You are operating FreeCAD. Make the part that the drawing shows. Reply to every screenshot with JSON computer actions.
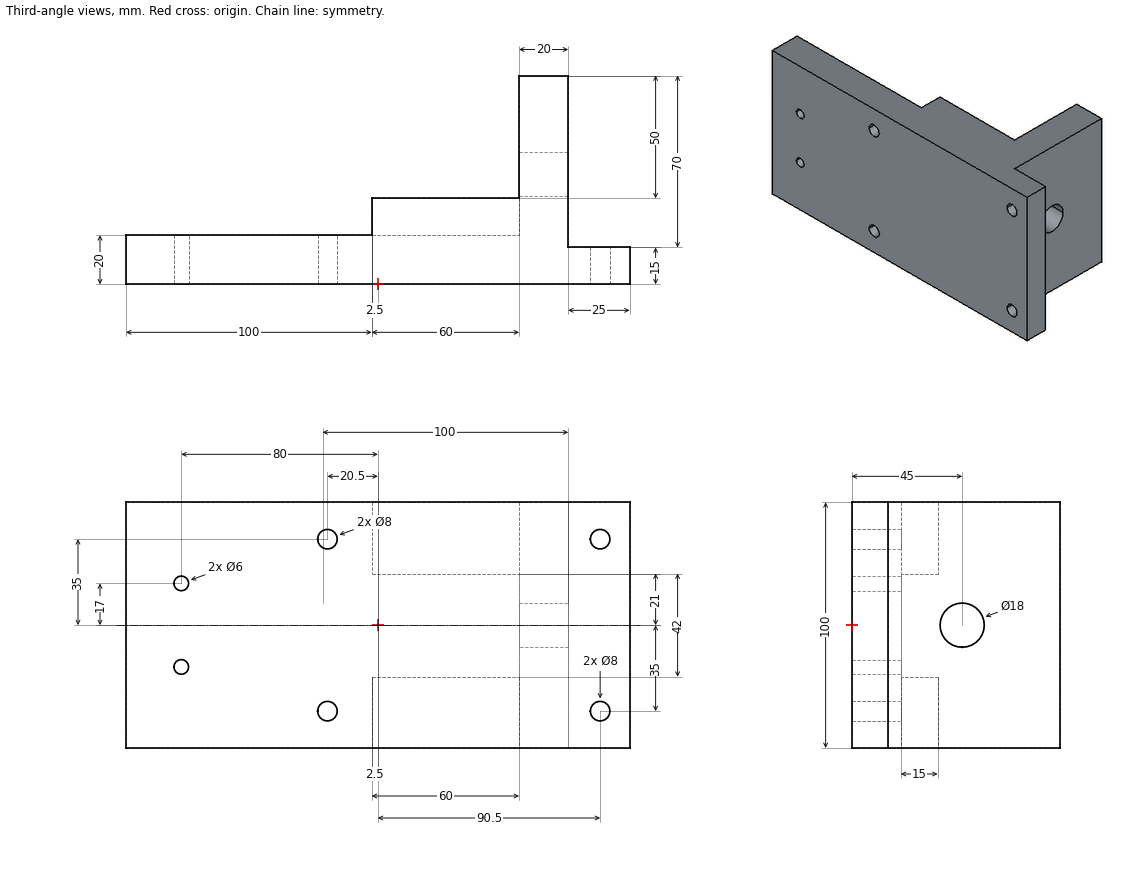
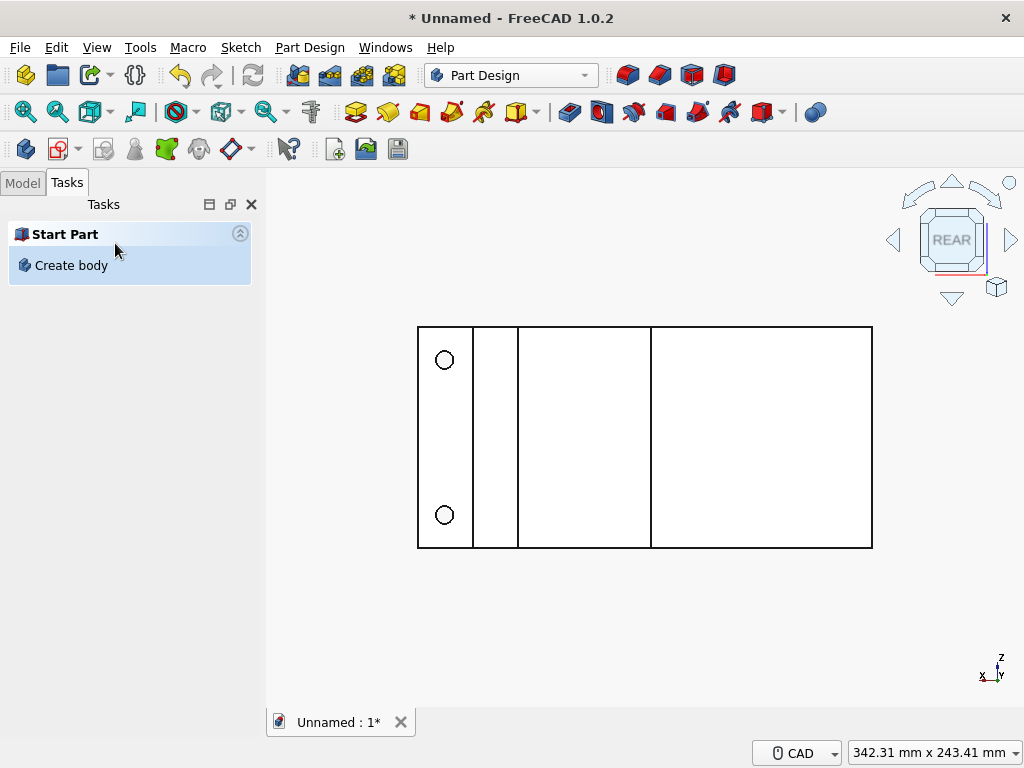
{"action": "left_click", "coordinate": [584, 405]}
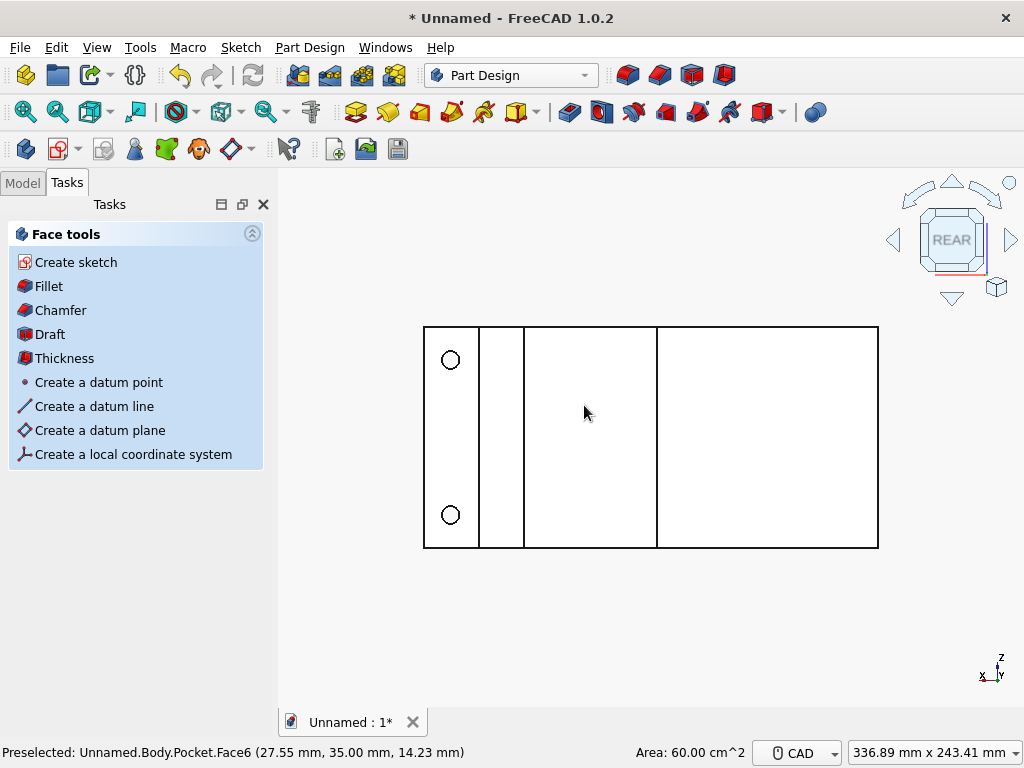
{"action": "left_click", "coordinate": [58, 150]}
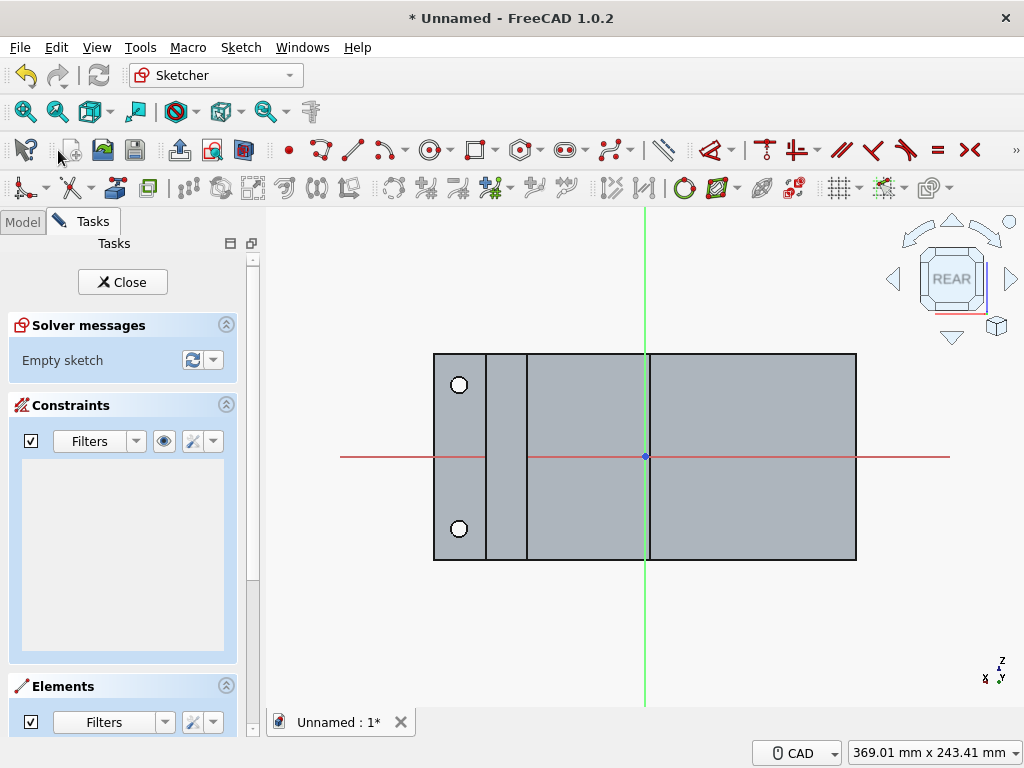
{"action": "left_click", "coordinate": [244, 150]}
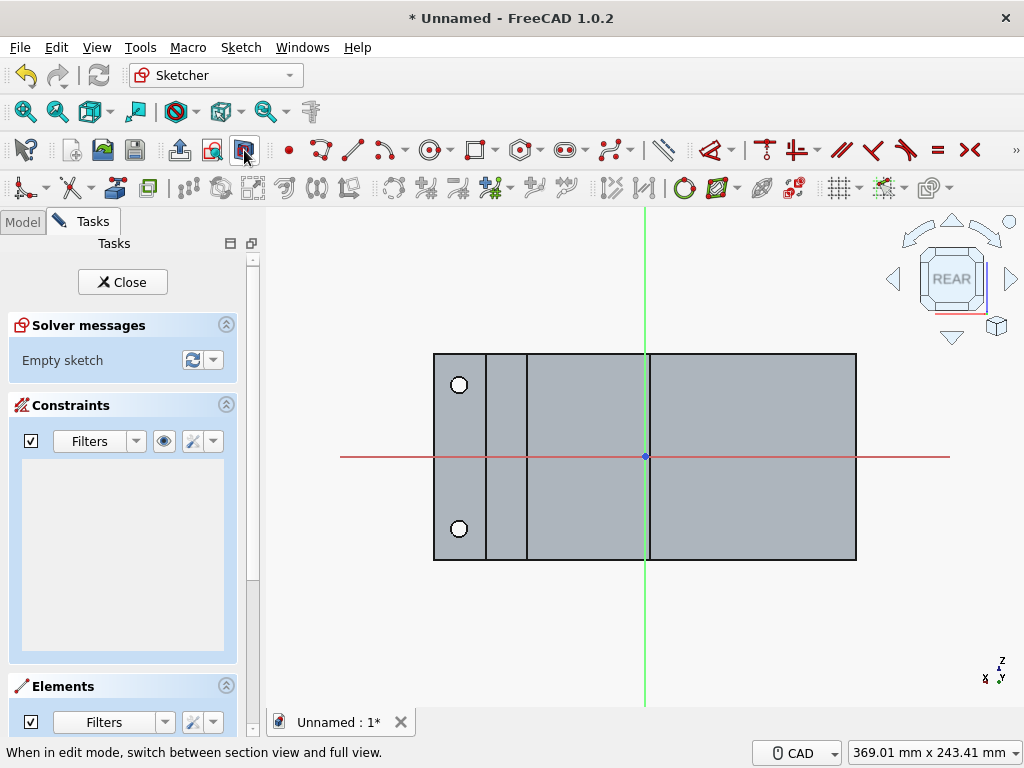
{"action": "scroll", "coordinate": [594, 457], "scroll_direction": "up", "scroll_amount": 6}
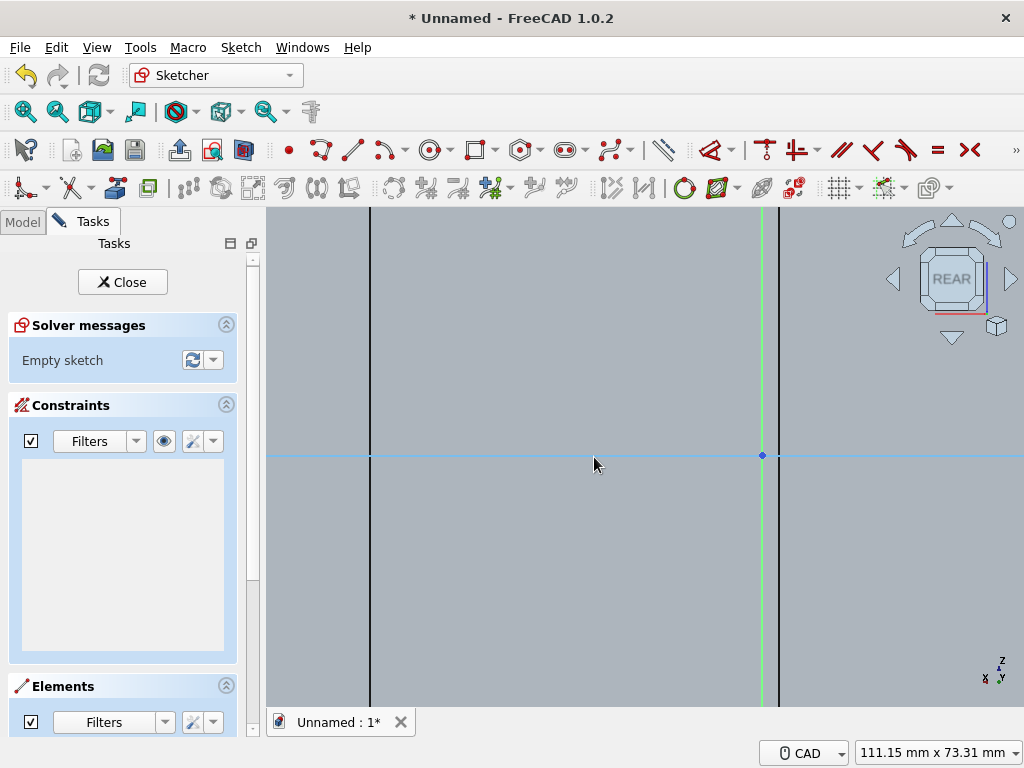
{"action": "left_click", "coordinate": [476, 150]}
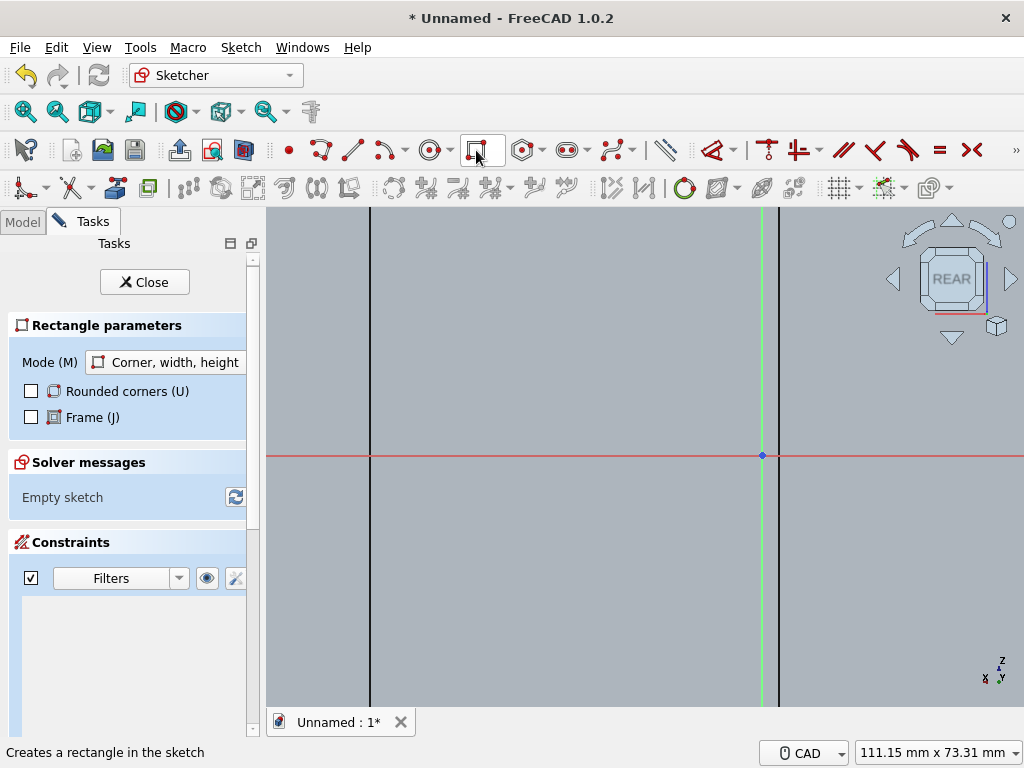
{"action": "left_click", "coordinate": [370, 313]}
{"action": "left_click", "coordinate": [779, 599]}
{"action": "key", "text": "Escape"}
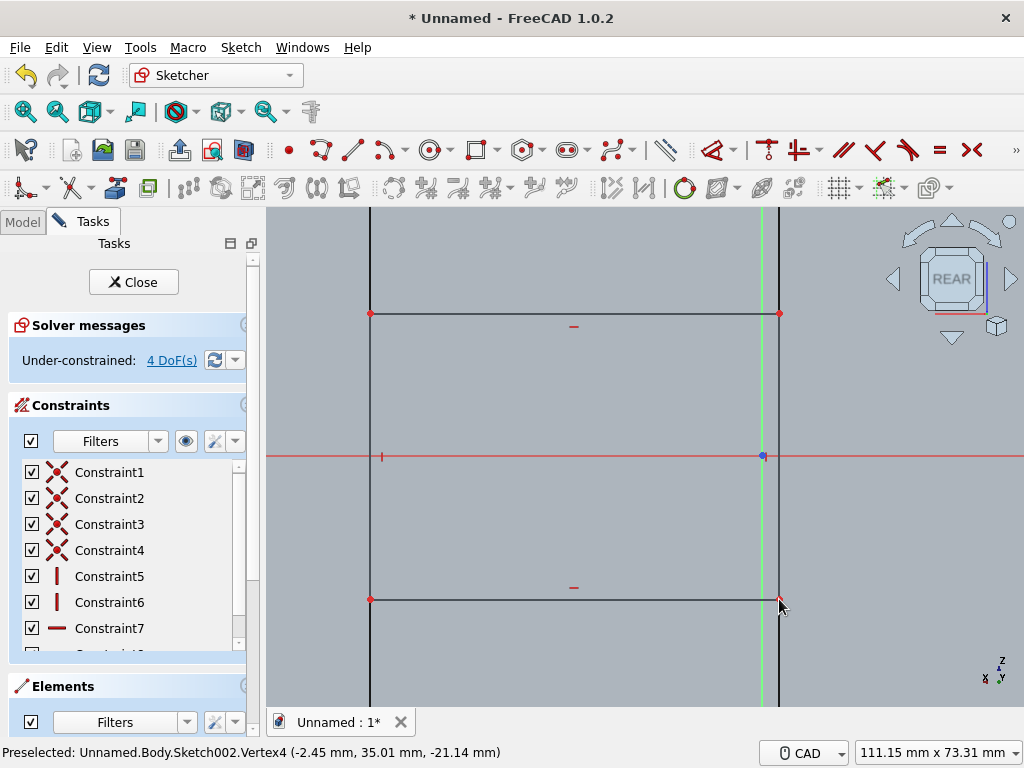
{"action": "left_click", "coordinate": [712, 150]}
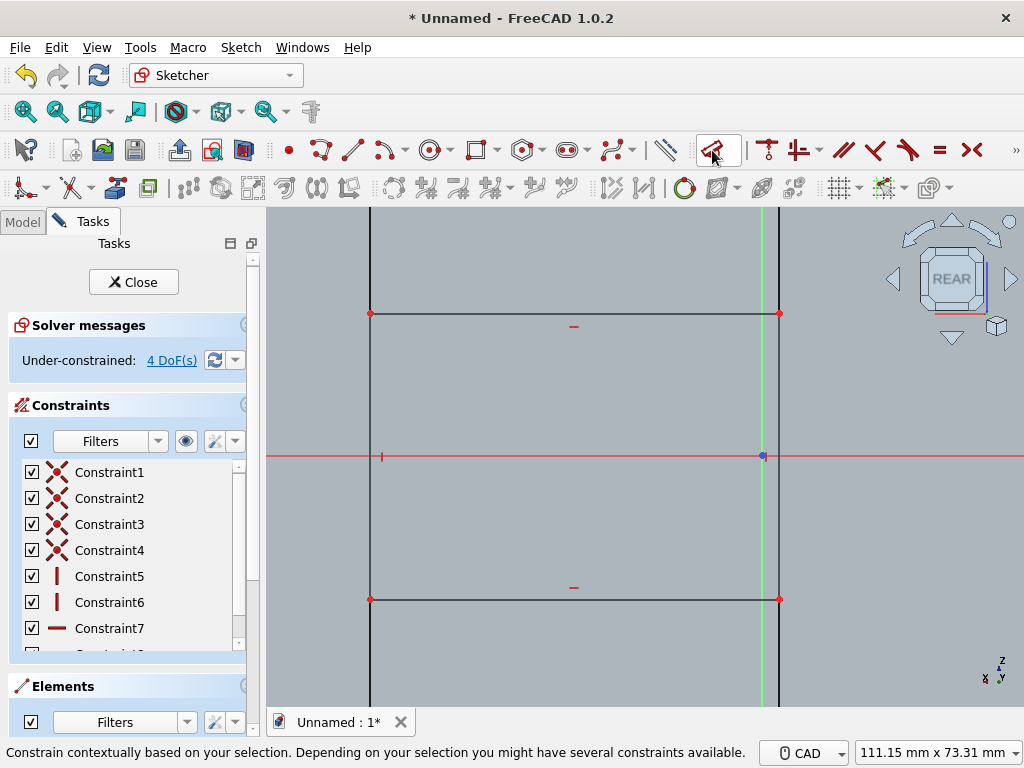
{"action": "left_click", "coordinate": [370, 400]}
{"action": "left_click", "coordinate": [336, 391]}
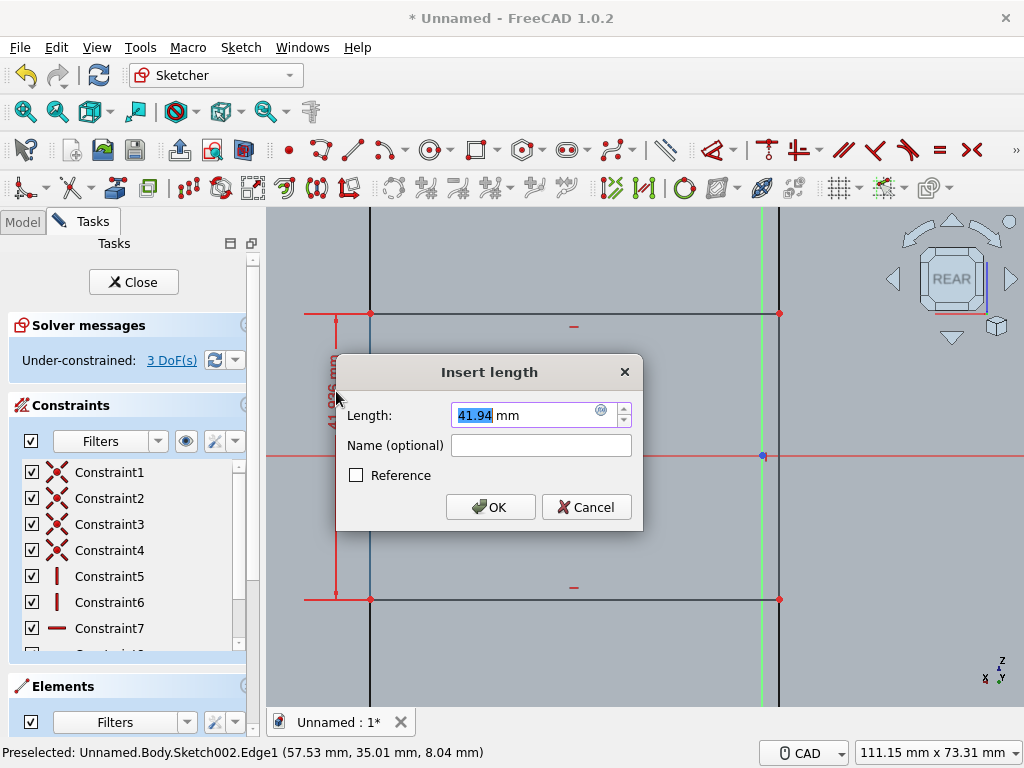
{"action": "type", "text": "42"}
{"action": "key", "text": "Return"}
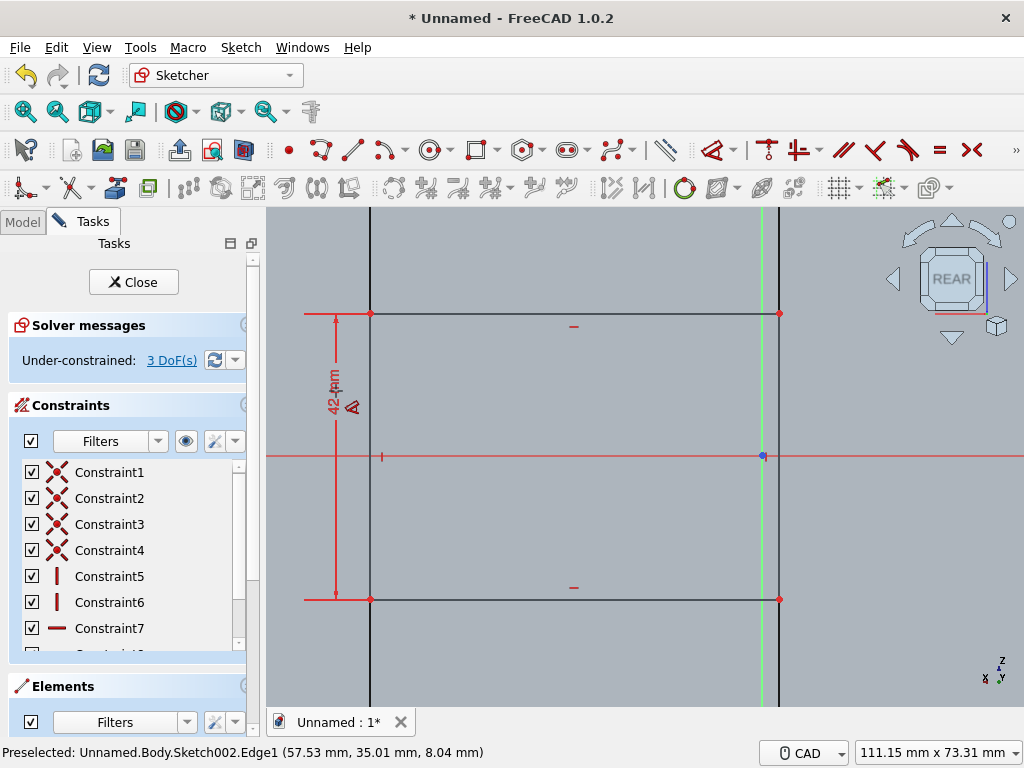
{"action": "left_click", "coordinate": [493, 600]}
{"action": "left_click", "coordinate": [575, 634]}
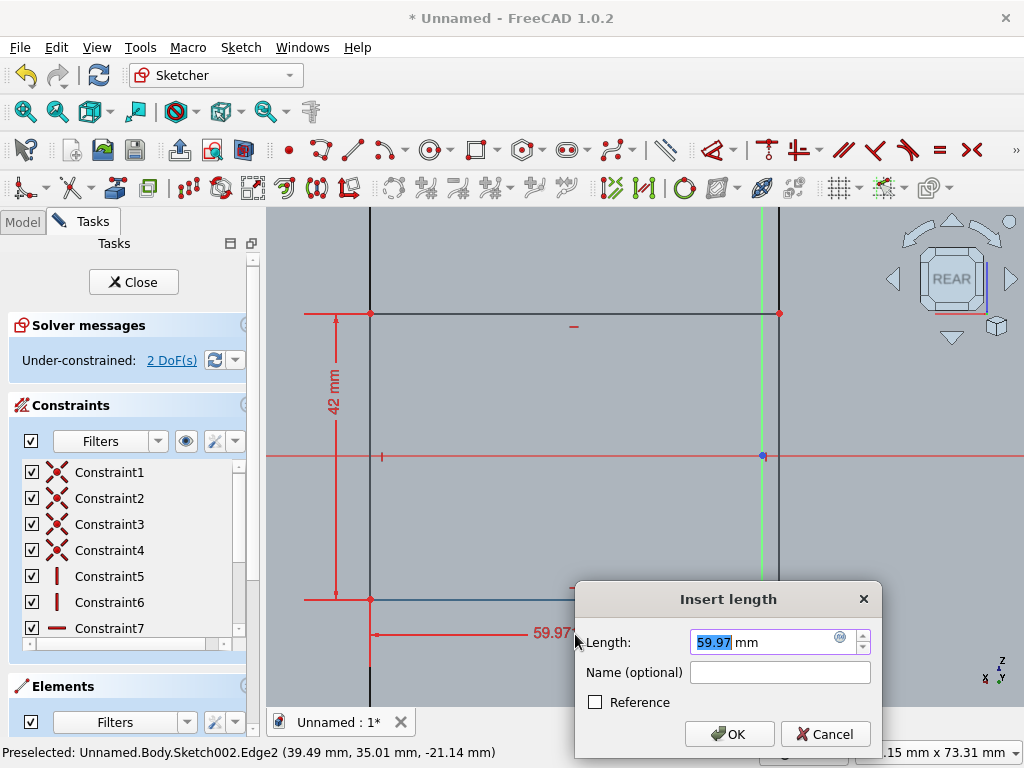
{"action": "type", "text": "60"}
{"action": "key", "text": "Return"}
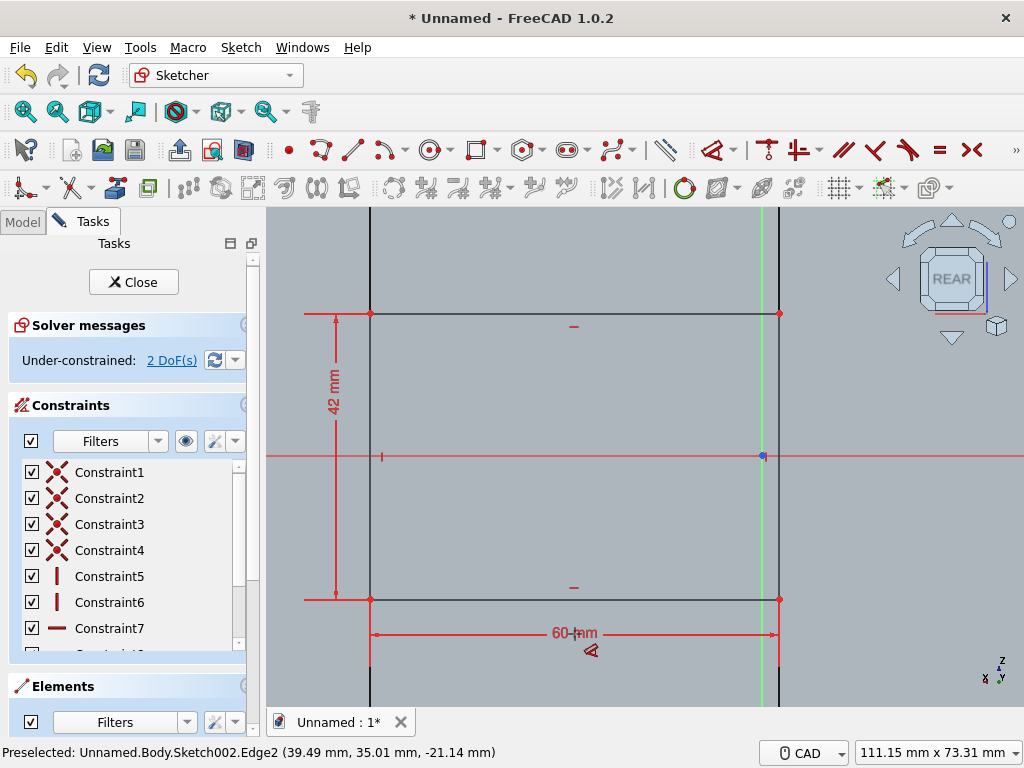
{"action": "left_click", "coordinate": [370, 314]}
{"action": "left_click", "coordinate": [336, 352]}